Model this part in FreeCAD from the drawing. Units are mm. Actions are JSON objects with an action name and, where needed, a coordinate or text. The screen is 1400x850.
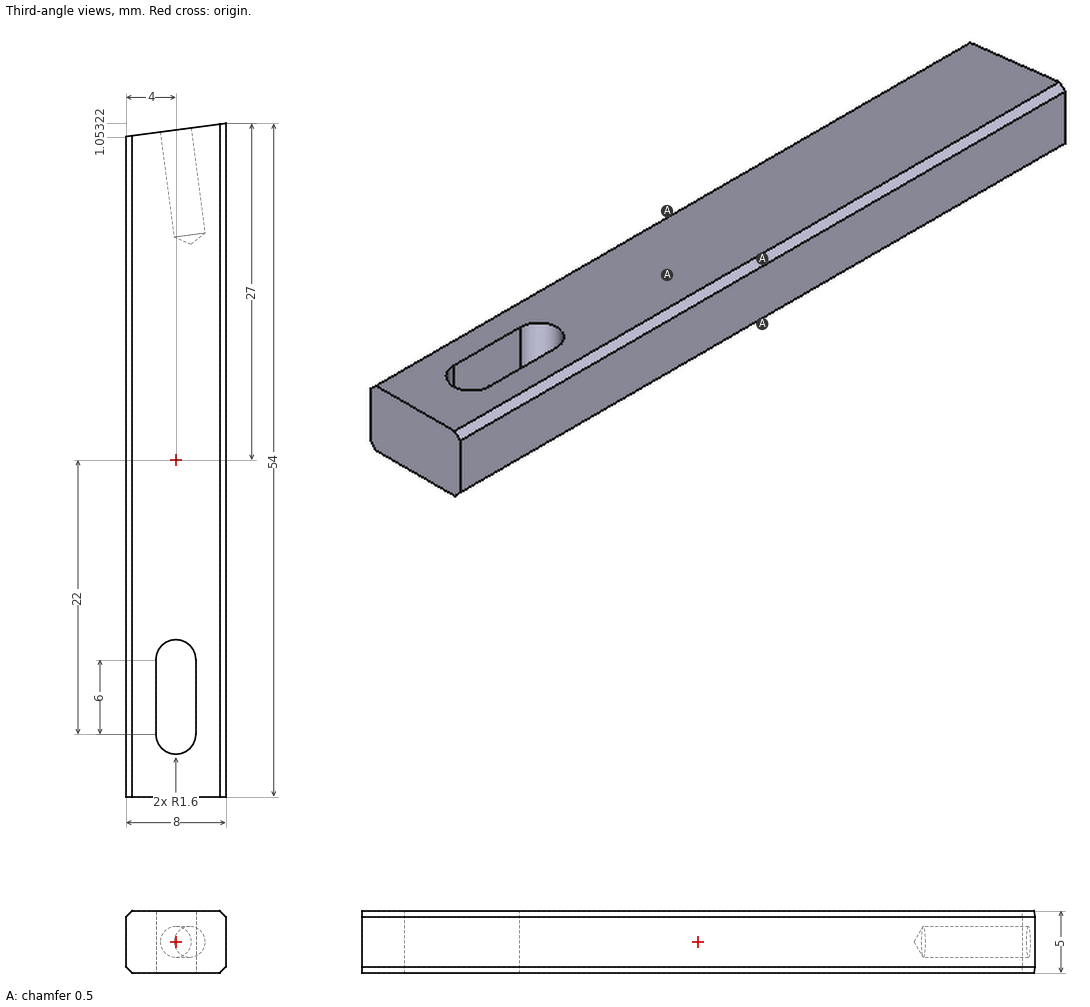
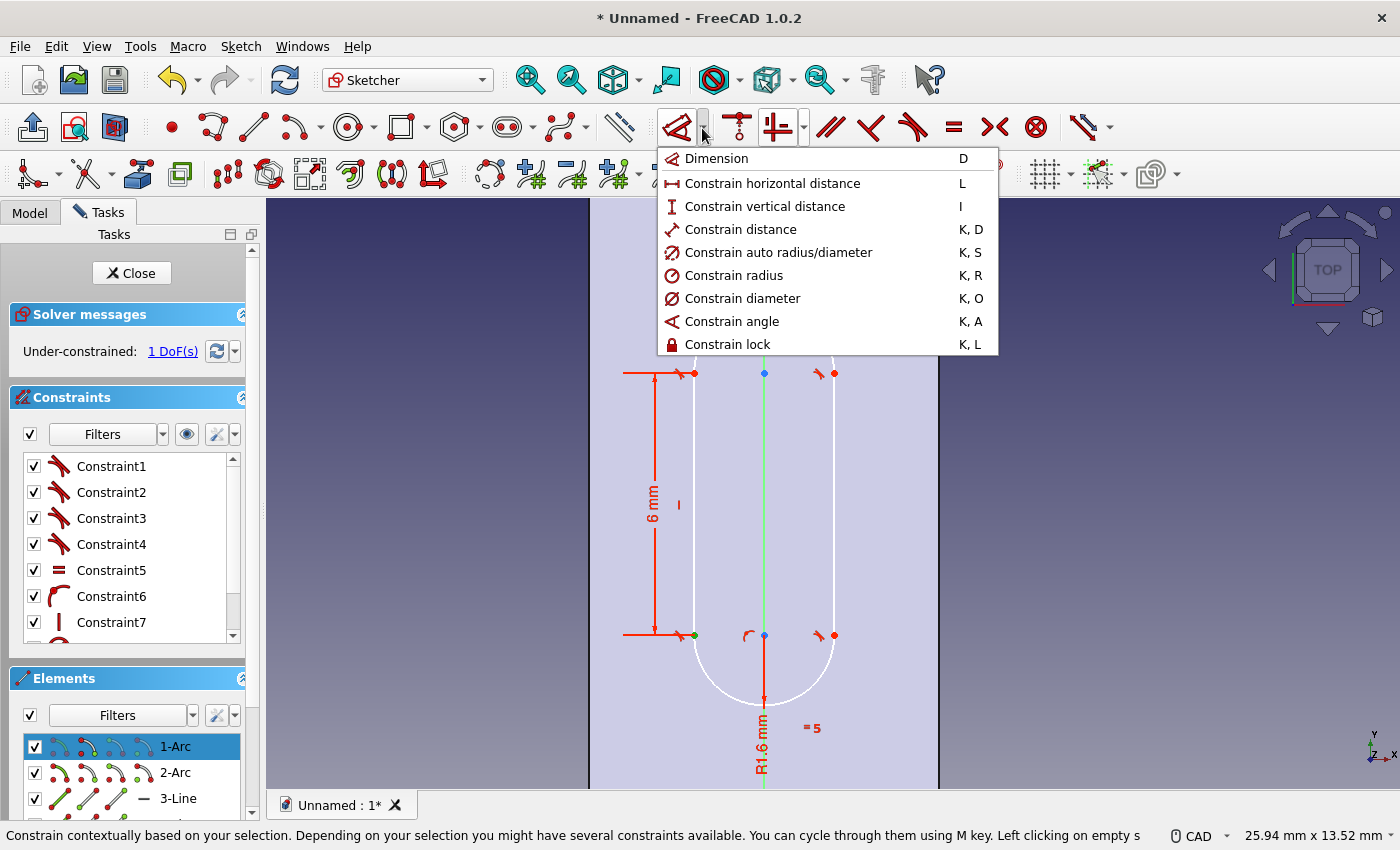
{"action": "left_click", "coordinate": [828, 206]}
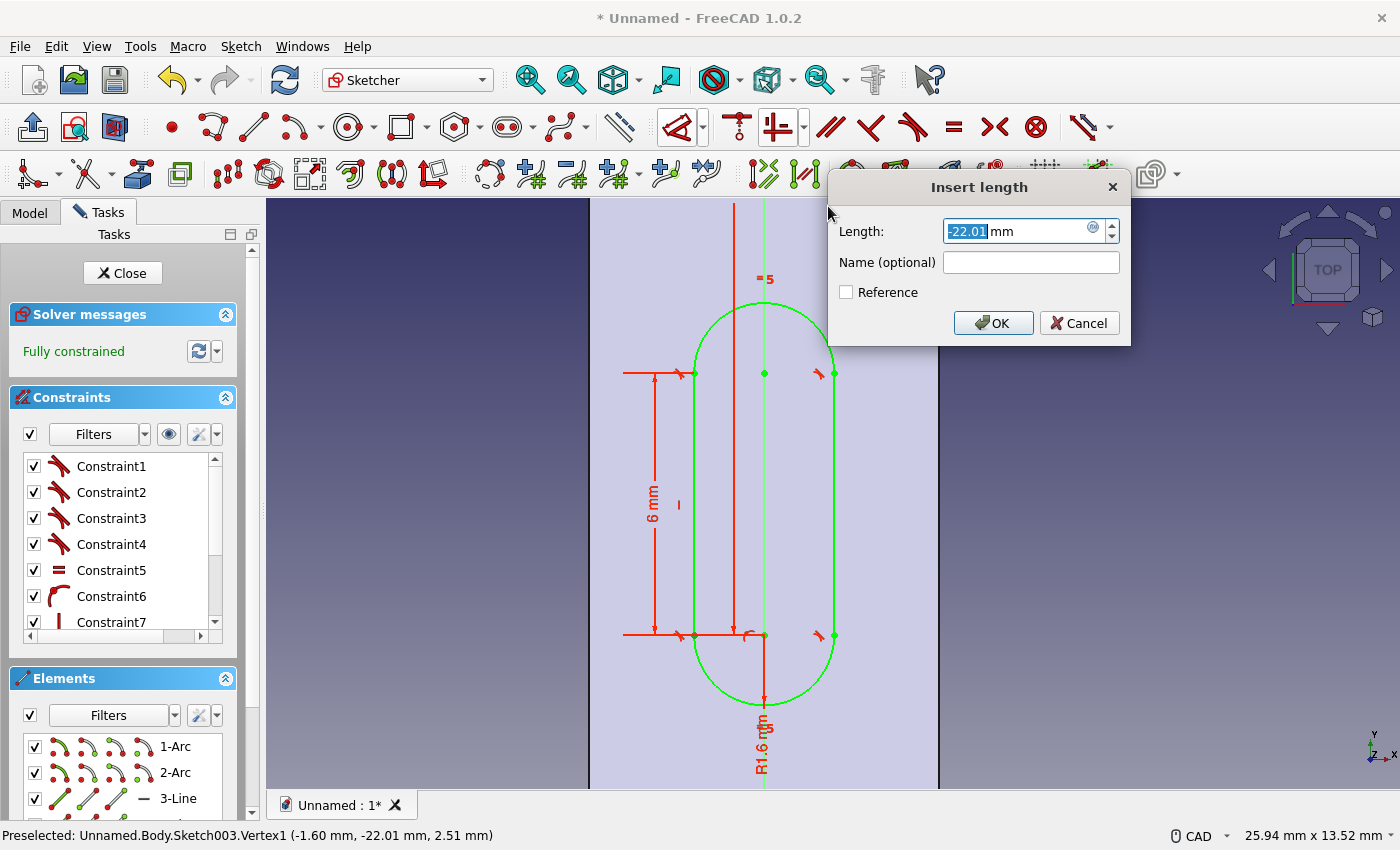
{"action": "type", "text": "-22"}
{"action": "key", "text": "Return"}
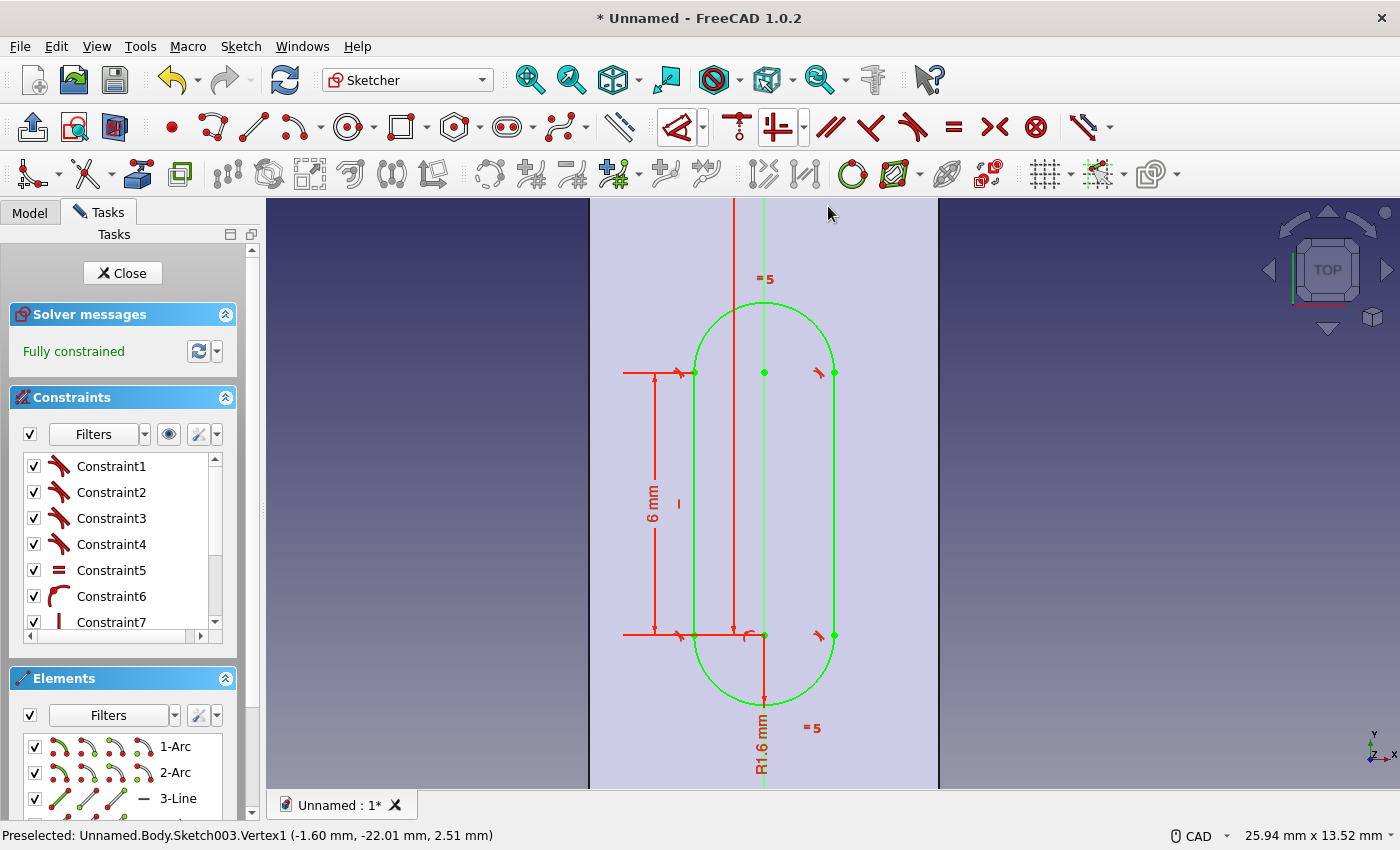
{"action": "left_click", "coordinate": [123, 273]}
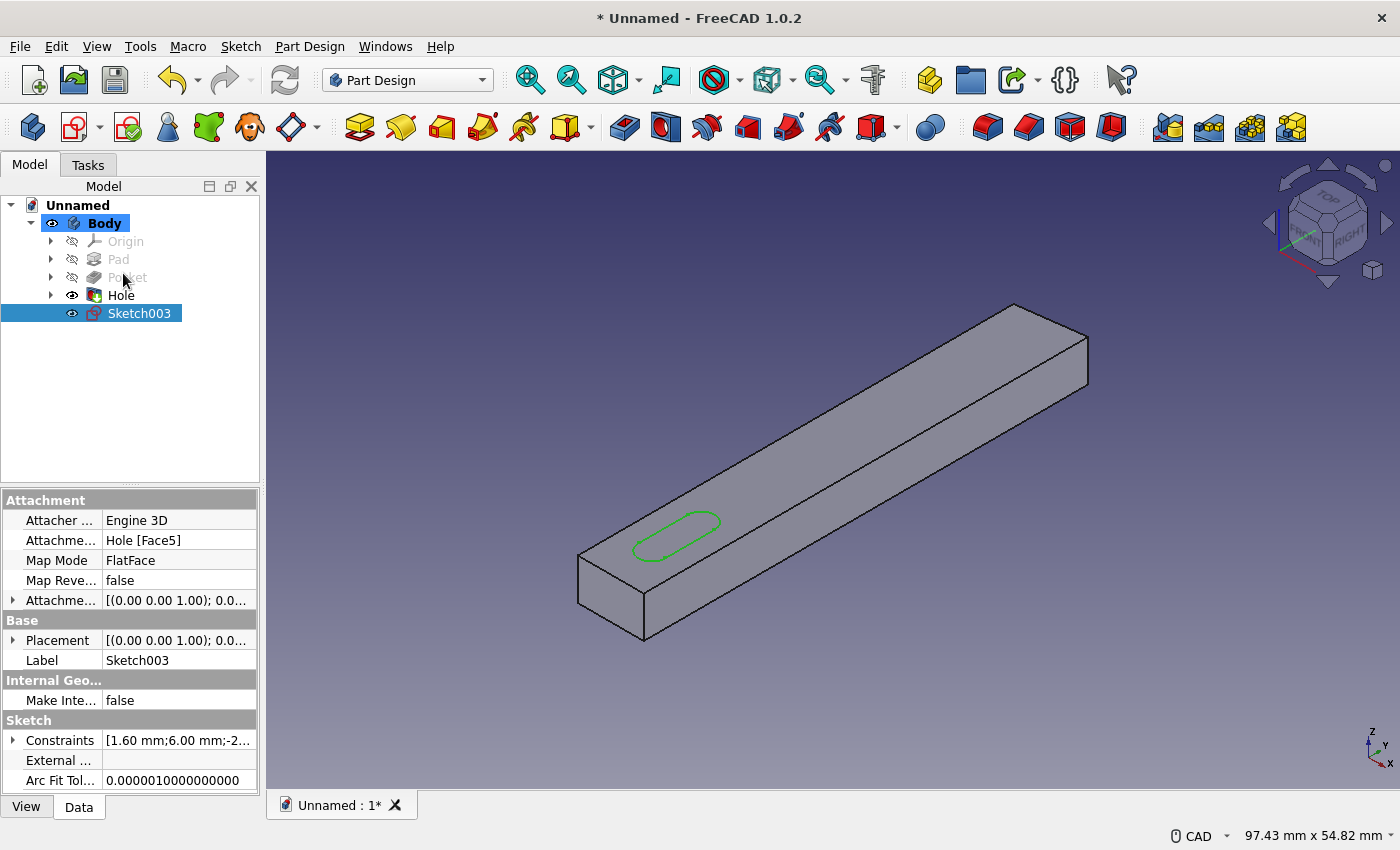
{"action": "left_click", "coordinate": [625, 128]}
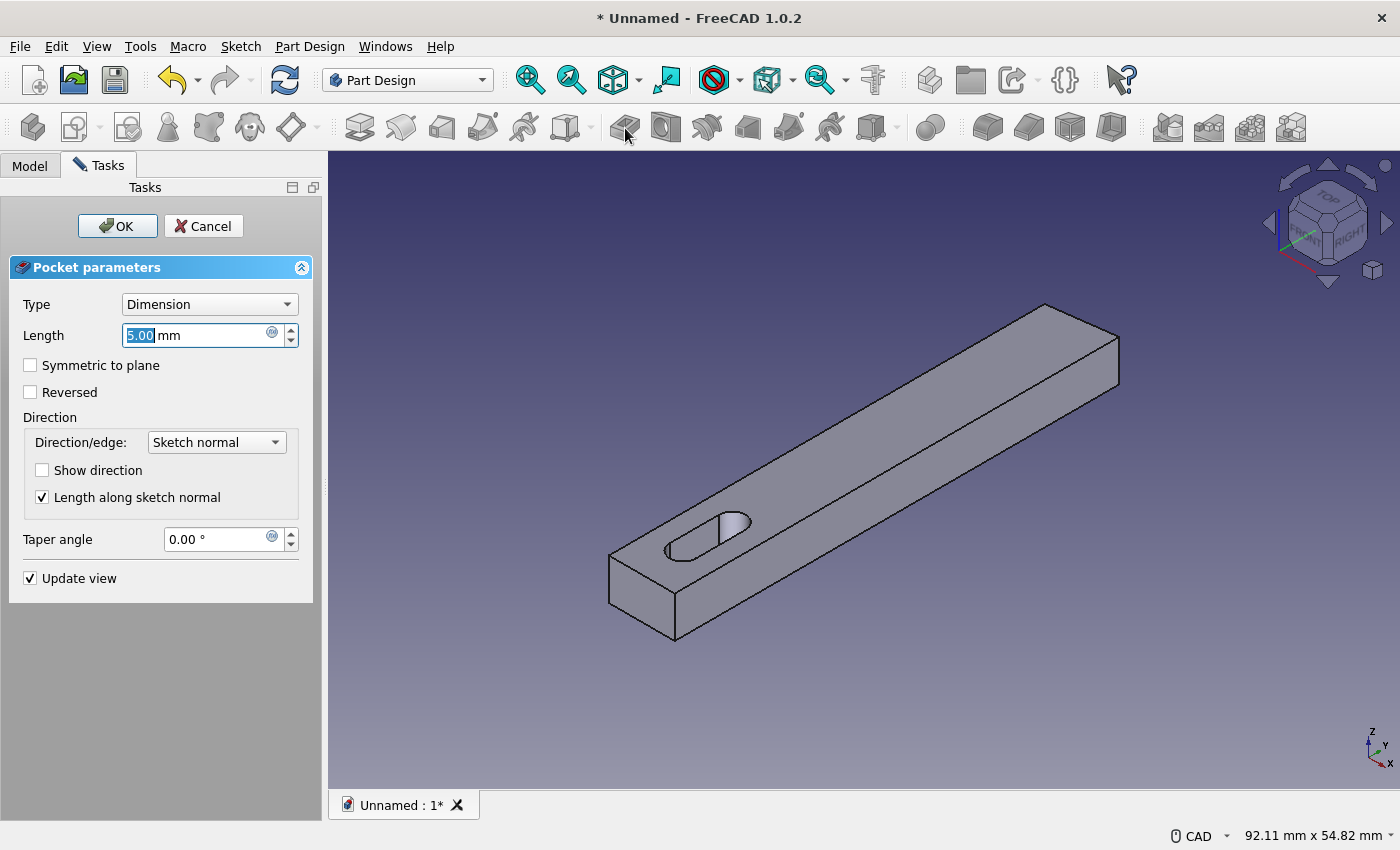
{"action": "left_click", "coordinate": [210, 304]}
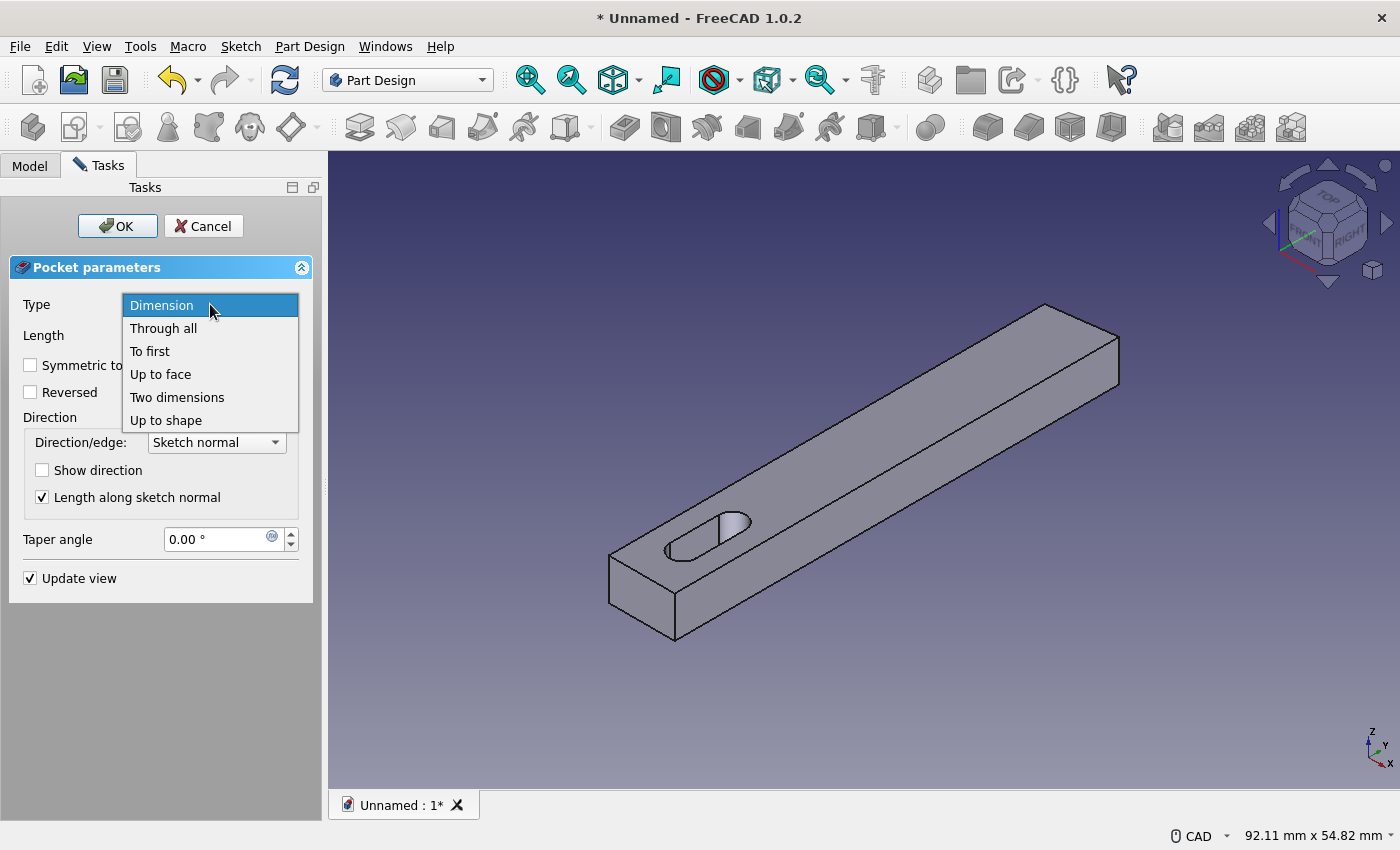
{"action": "left_click", "coordinate": [208, 328]}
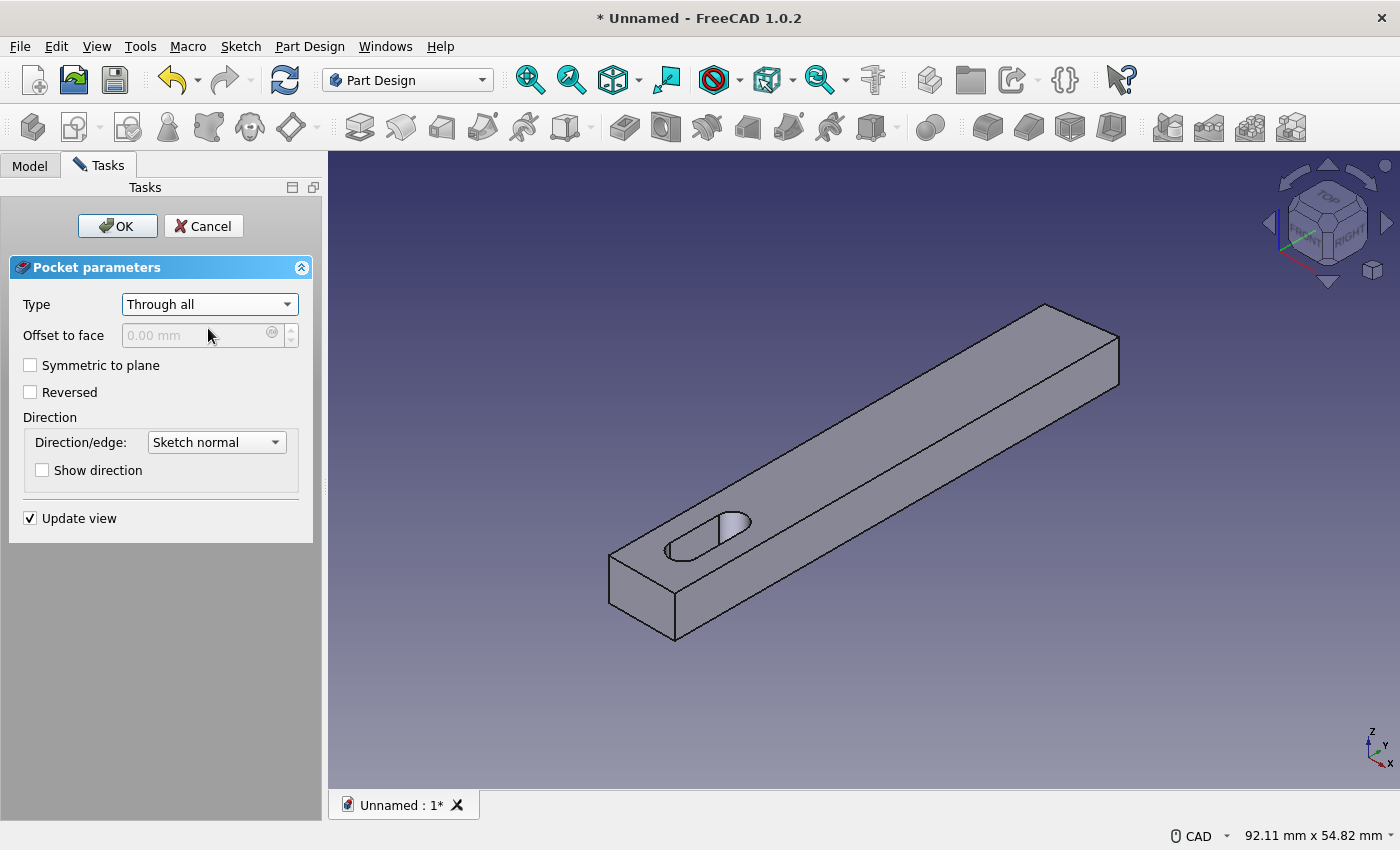
{"action": "left_click", "coordinate": [118, 226]}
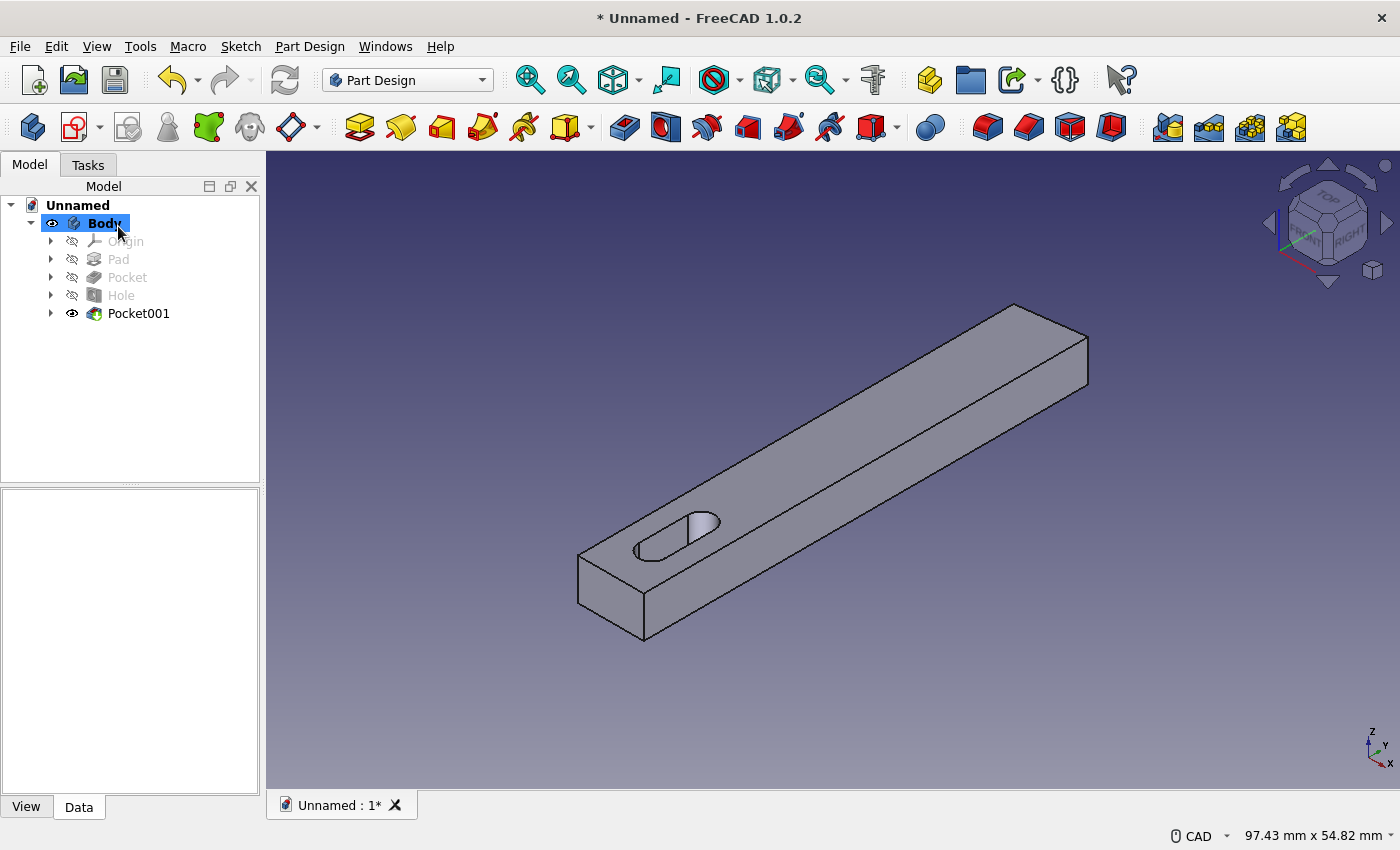
{"action": "left_click", "coordinate": [866, 464]}